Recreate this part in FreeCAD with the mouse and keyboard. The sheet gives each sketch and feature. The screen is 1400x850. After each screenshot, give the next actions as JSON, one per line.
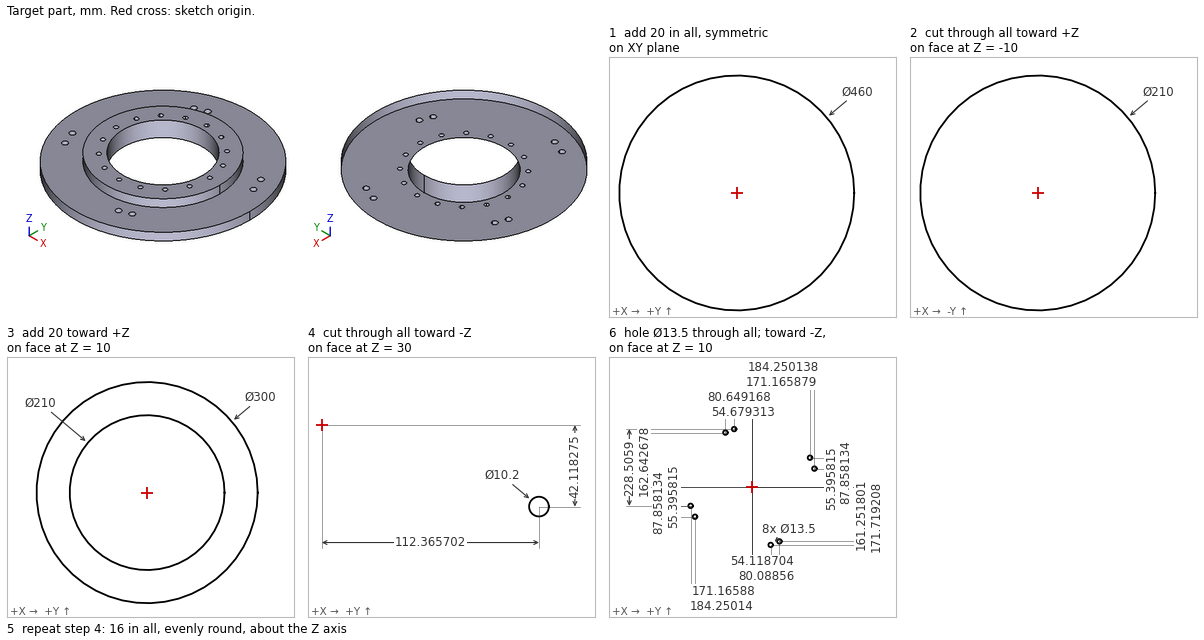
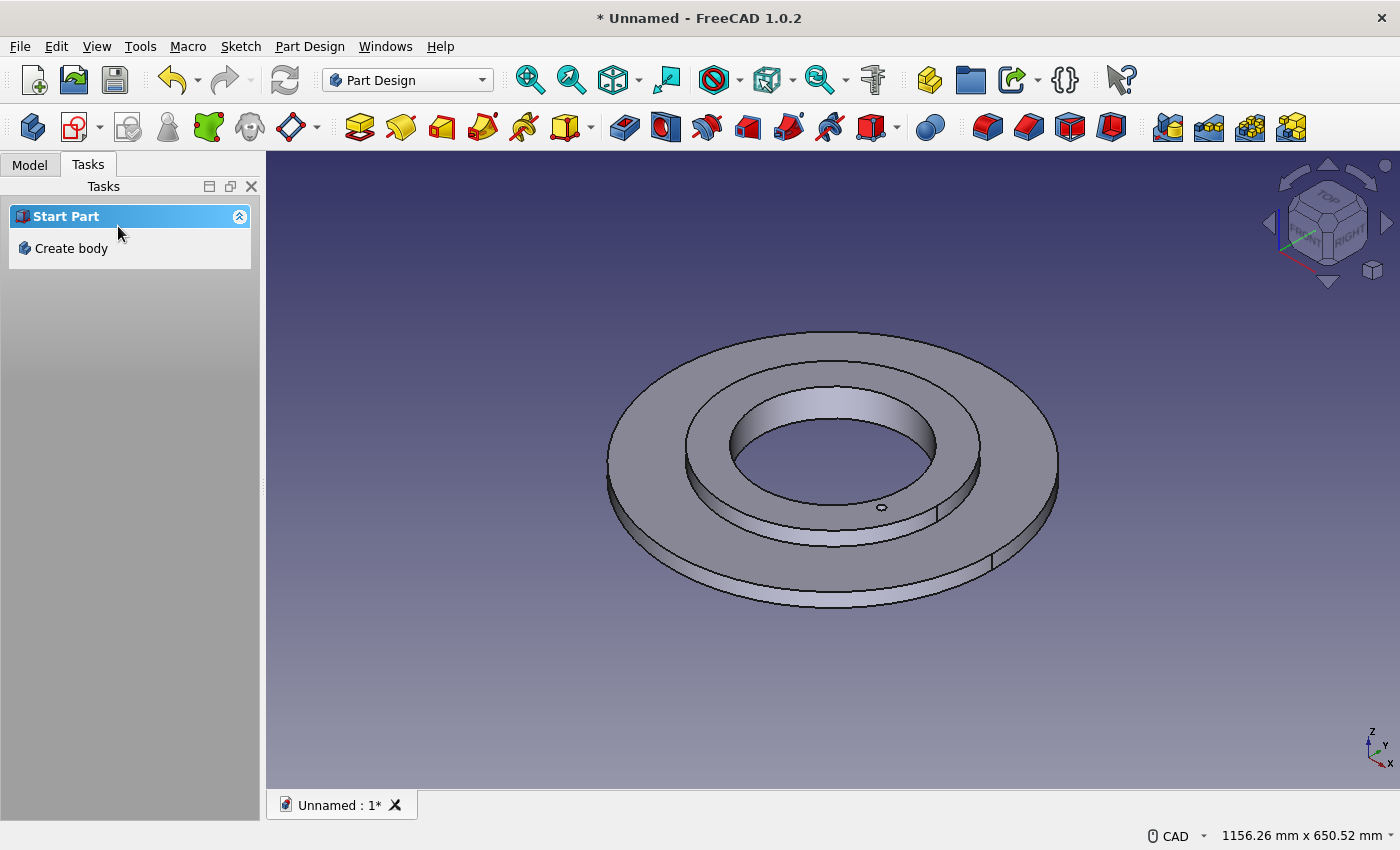
{"action": "left_click", "coordinate": [30, 164]}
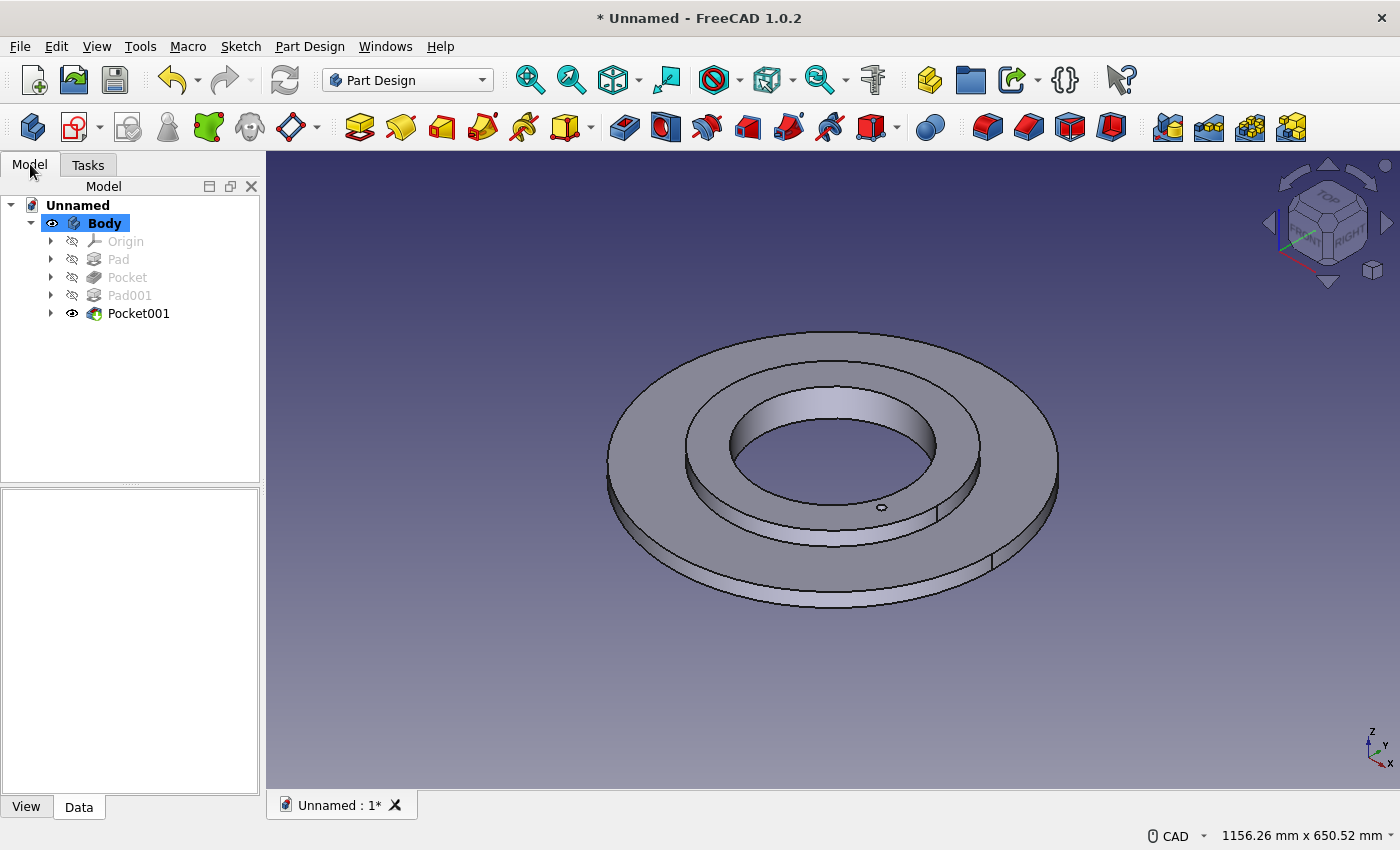
{"action": "left_click", "coordinate": [117, 313]}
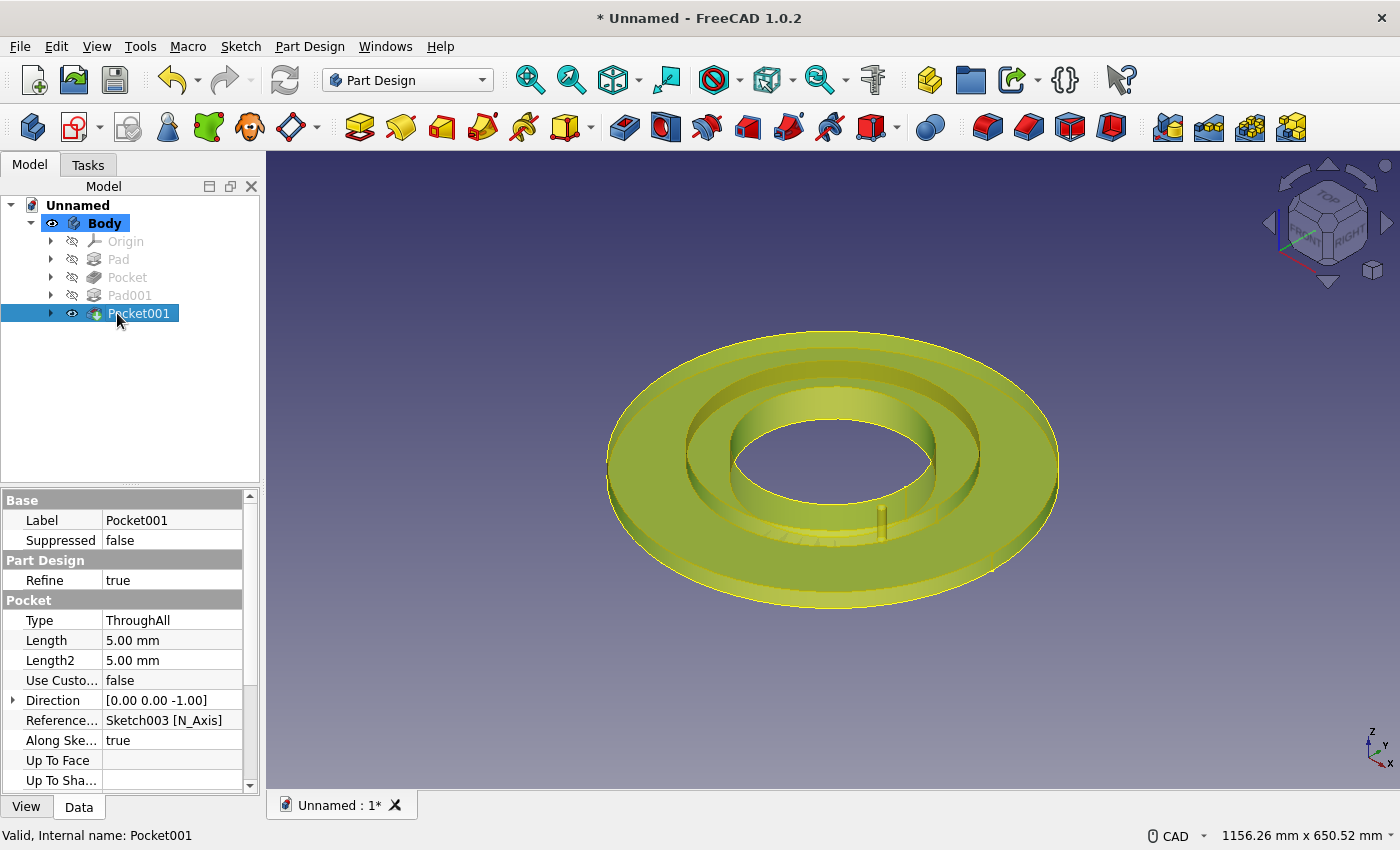
{"action": "left_click", "coordinate": [1250, 128]}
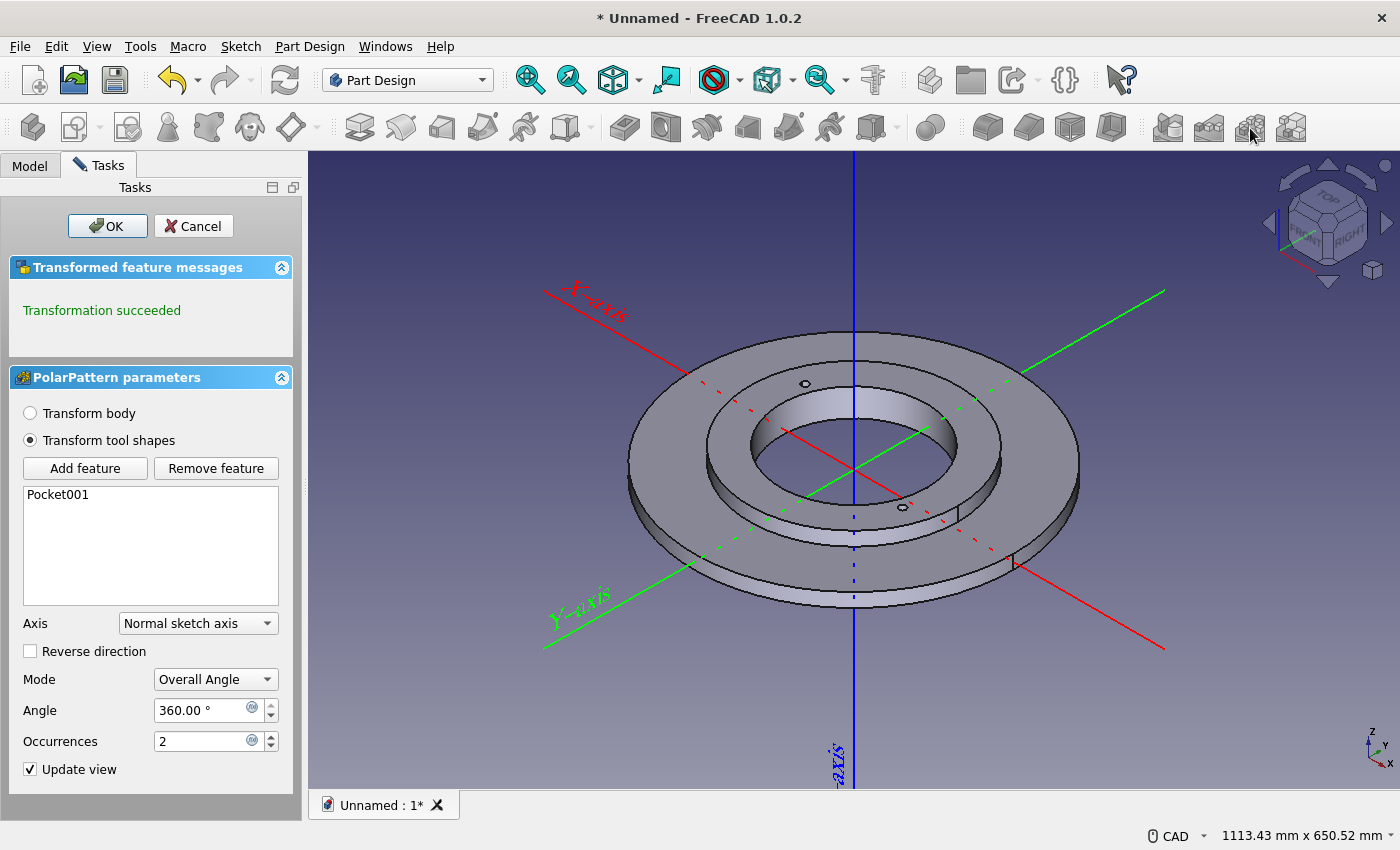
{"action": "left_click", "coordinate": [199, 624]}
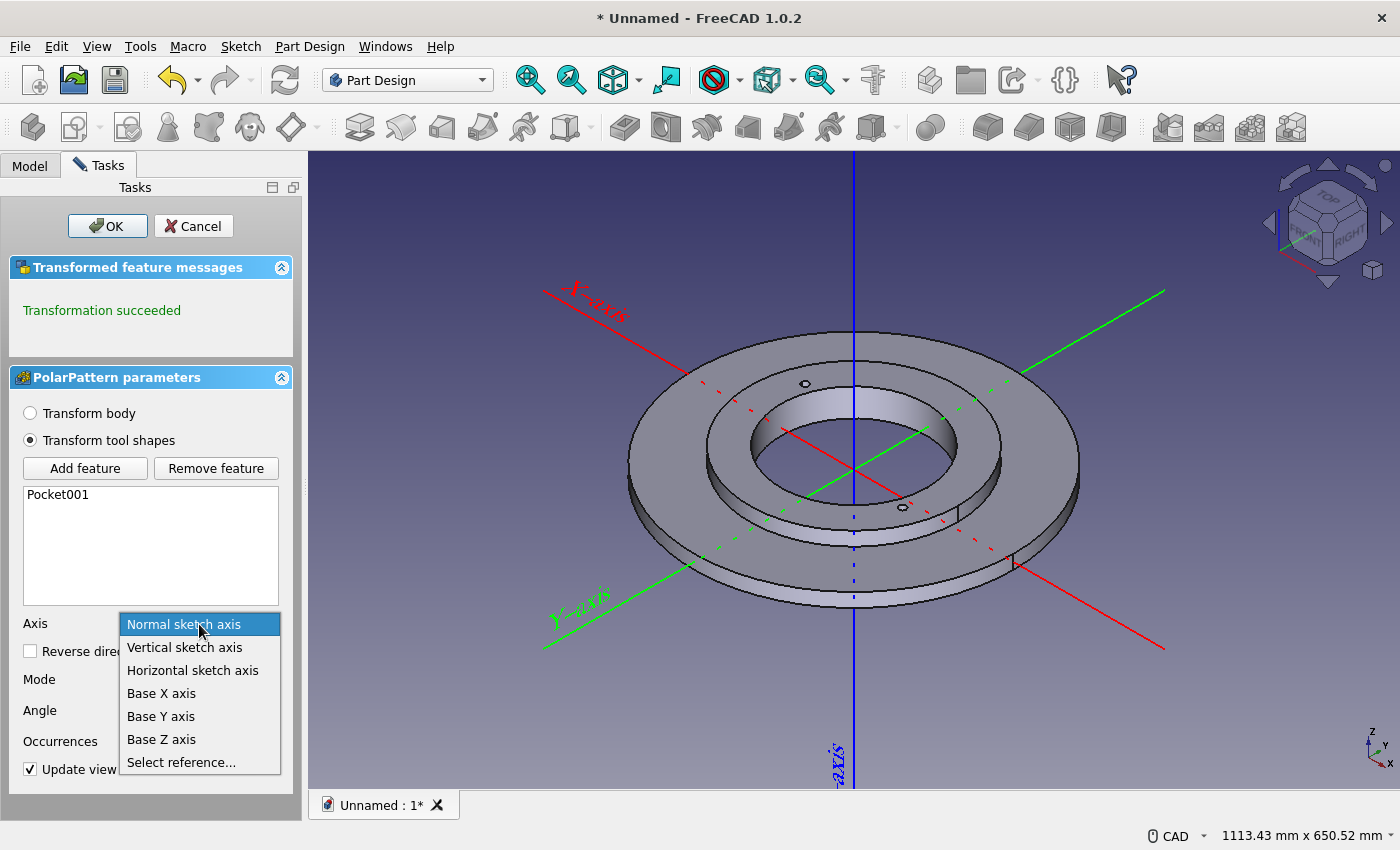
{"action": "left_click", "coordinate": [198, 740]}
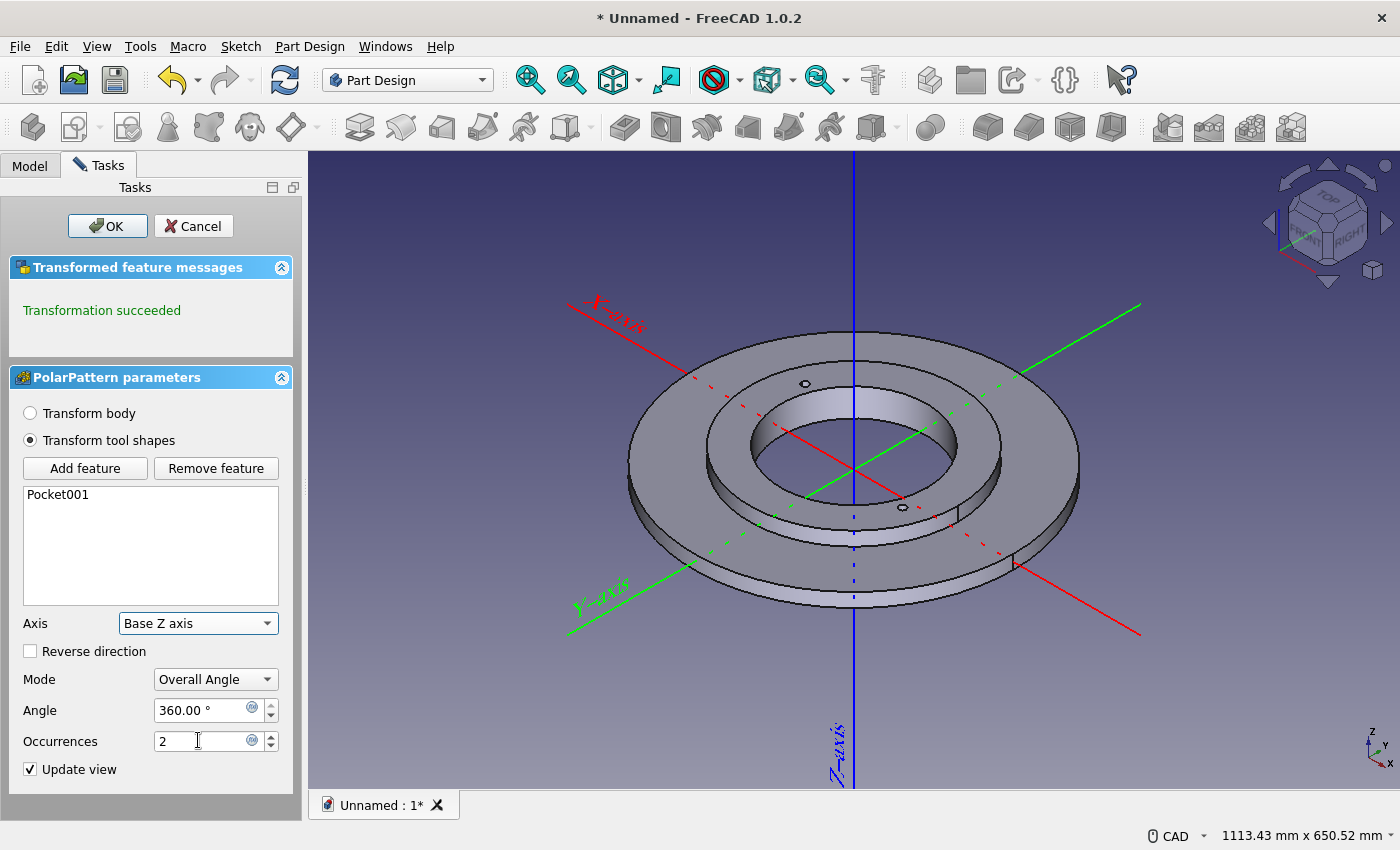
{"action": "triple_click", "coordinate": [210, 742]}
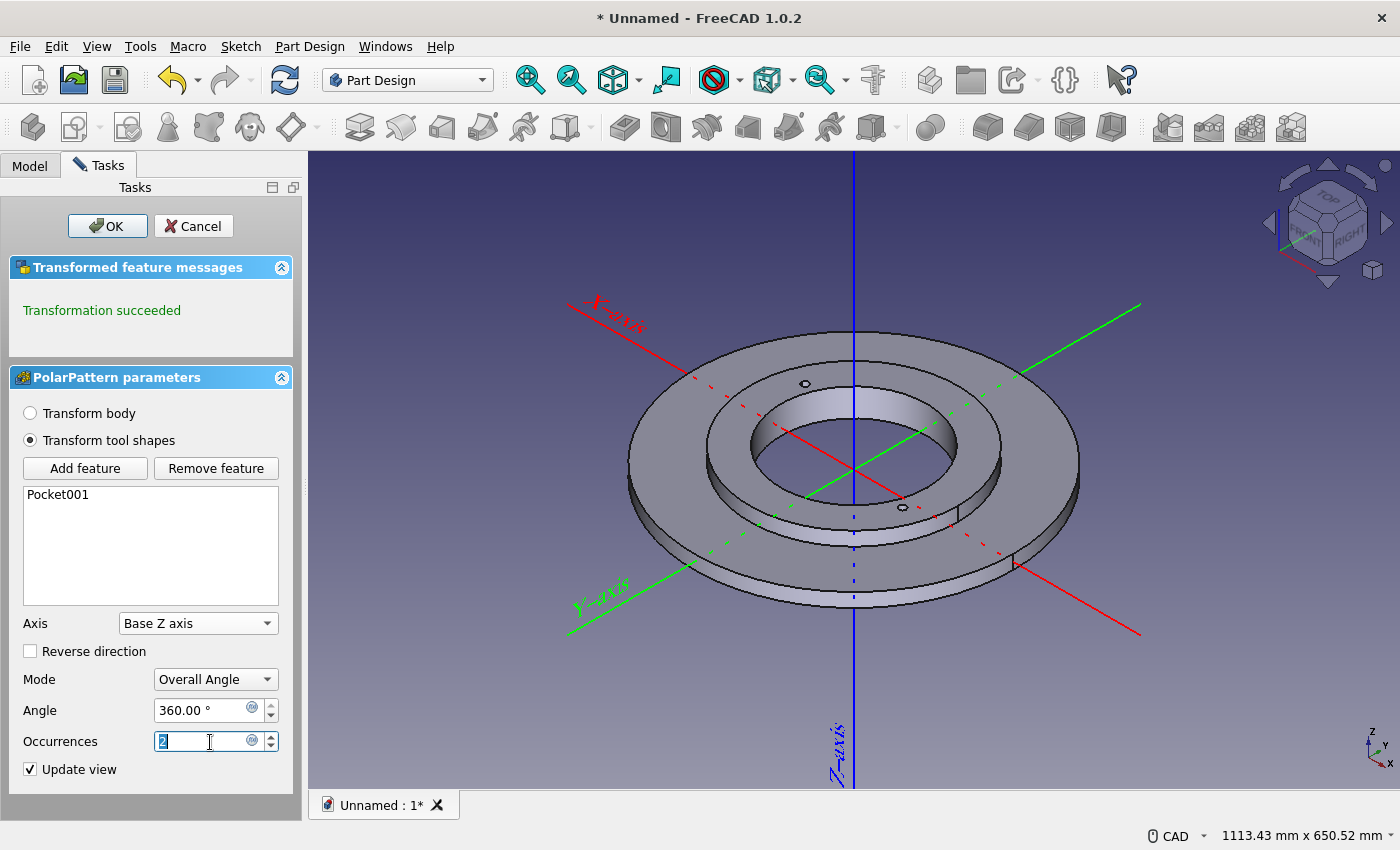
{"action": "type", "text": "16"}
{"action": "key", "text": "Tab"}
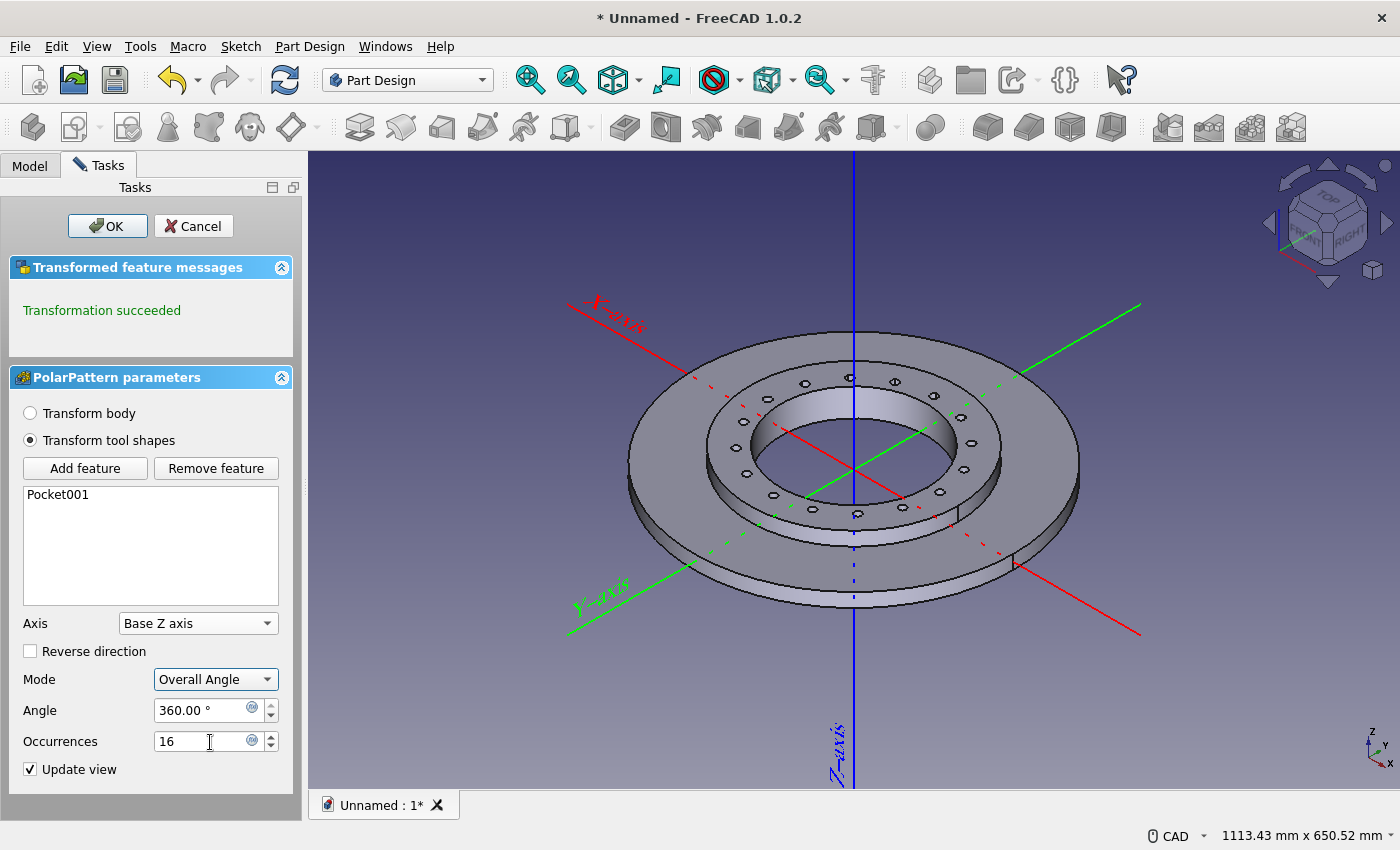
{"action": "left_click", "coordinate": [108, 226]}